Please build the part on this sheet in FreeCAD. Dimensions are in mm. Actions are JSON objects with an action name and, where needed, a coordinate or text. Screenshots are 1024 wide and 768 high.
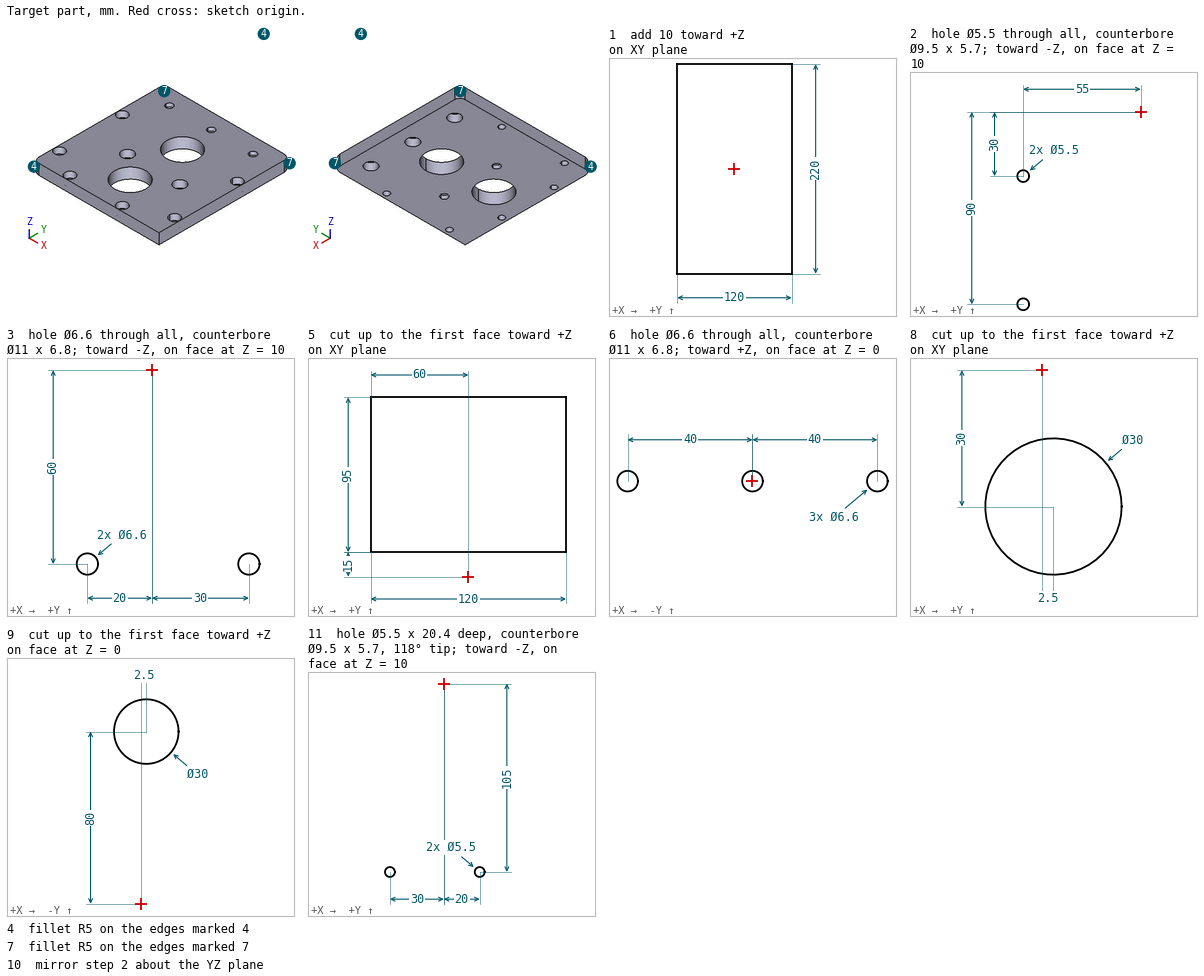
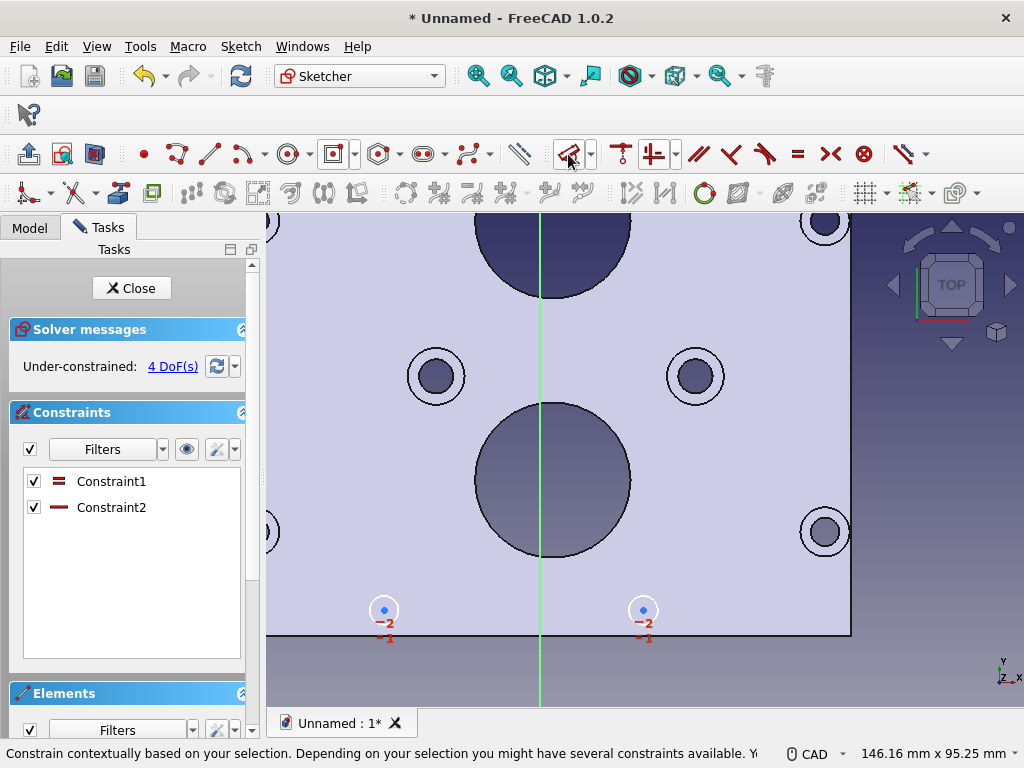
{"action": "scroll", "coordinate": [653, 600], "scroll_direction": "up", "scroll_amount": 2}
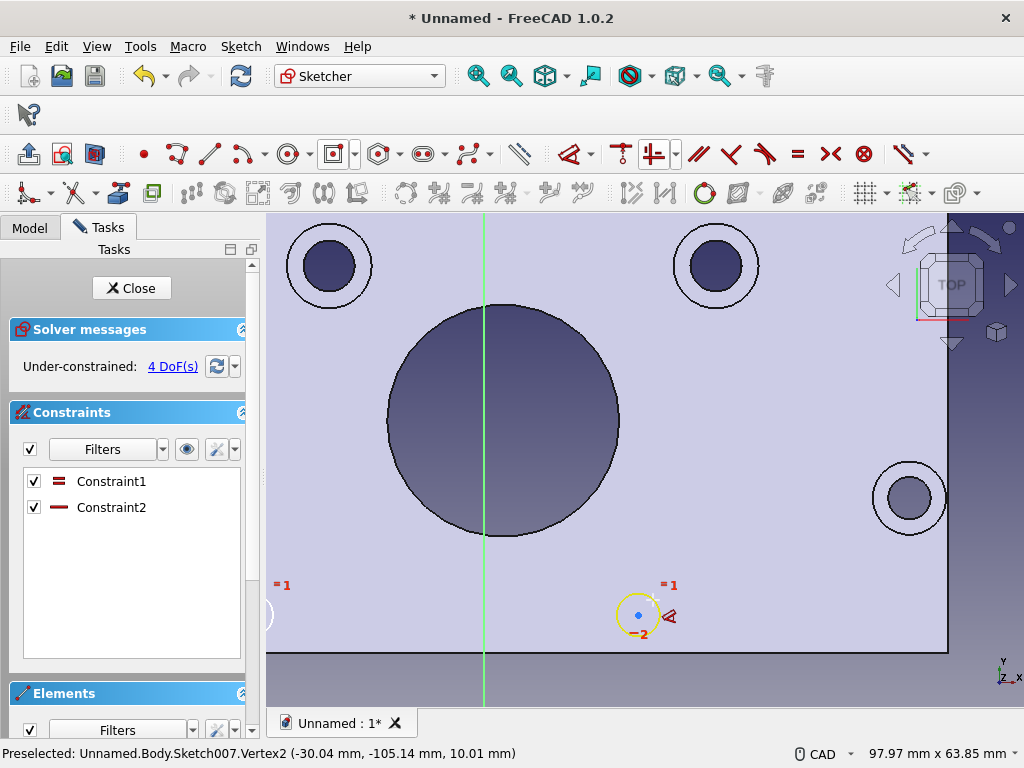
{"action": "left_click", "coordinate": [653, 600]}
{"action": "left_click", "coordinate": [675, 577]}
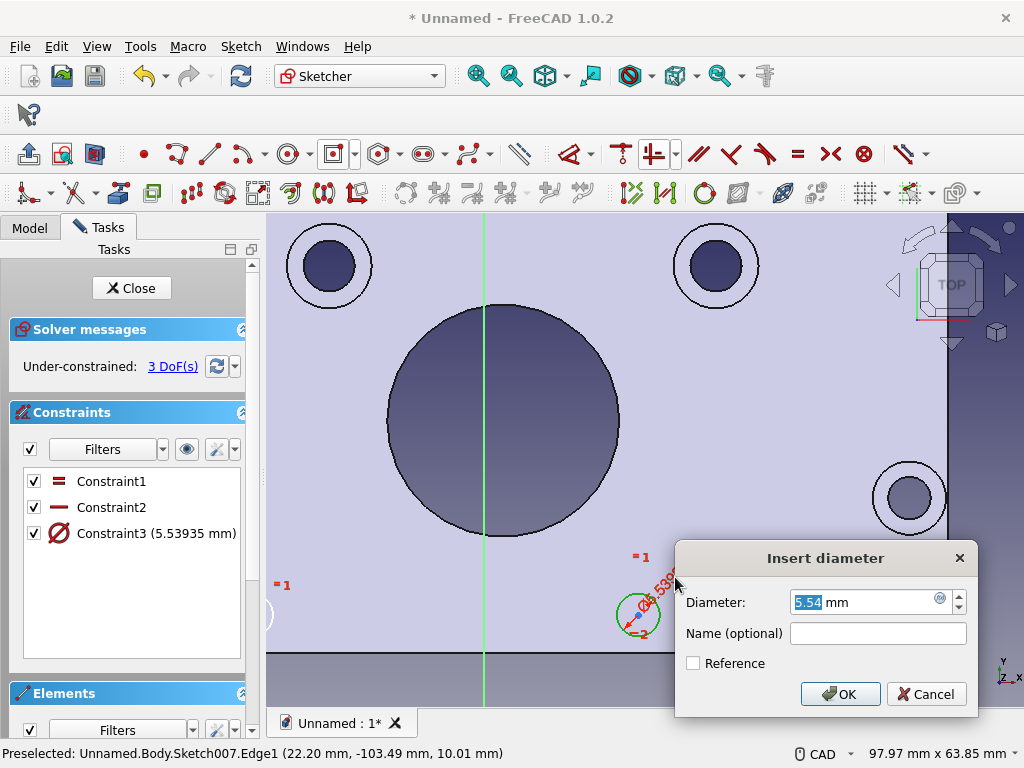
{"action": "type", "text": "5.5"}
{"action": "key", "text": "Return"}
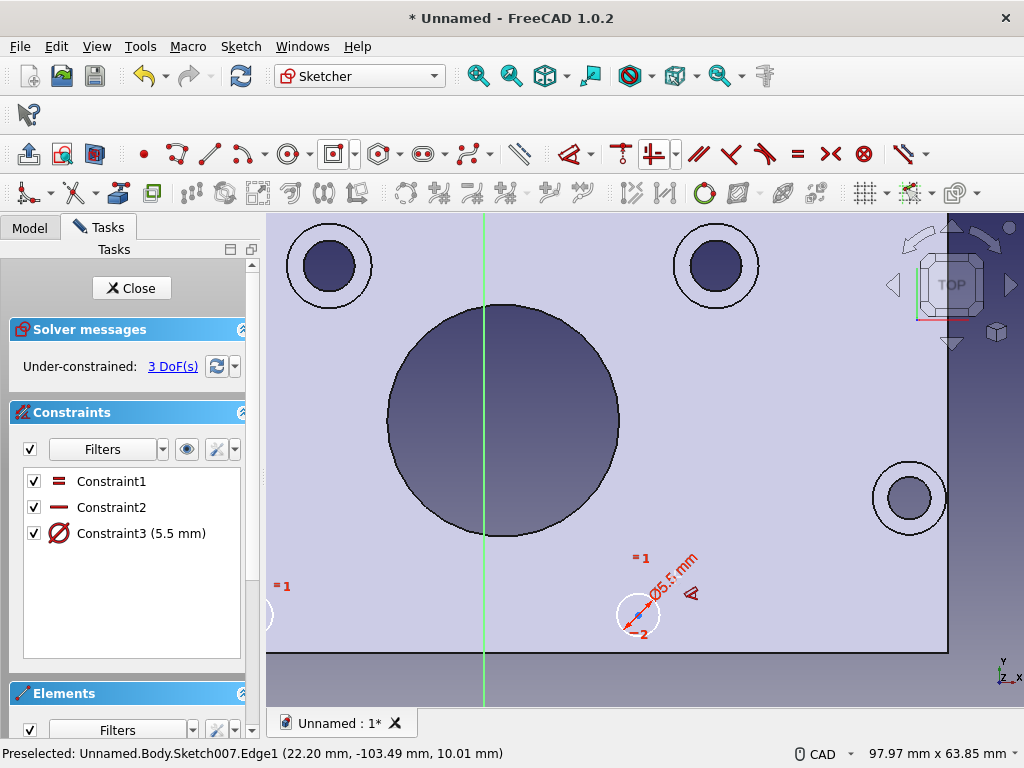
{"action": "left_click", "coordinate": [638, 615]}
{"action": "left_click", "coordinate": [561, 649]}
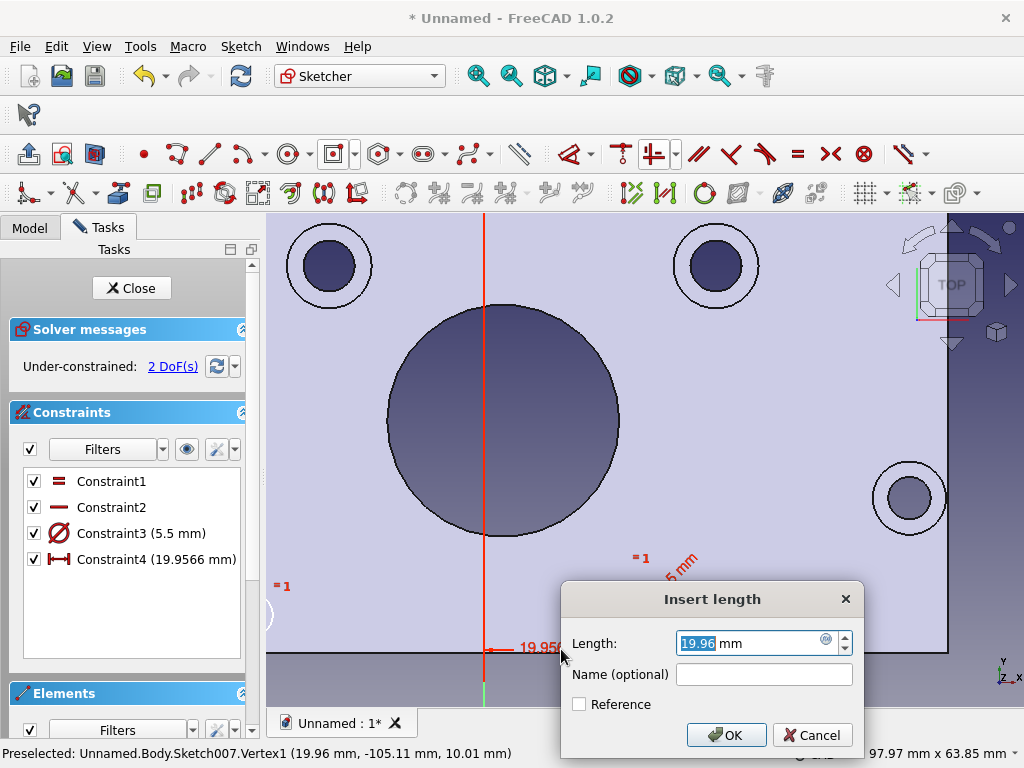
{"action": "type", "text": "20"}
{"action": "key", "text": "Return"}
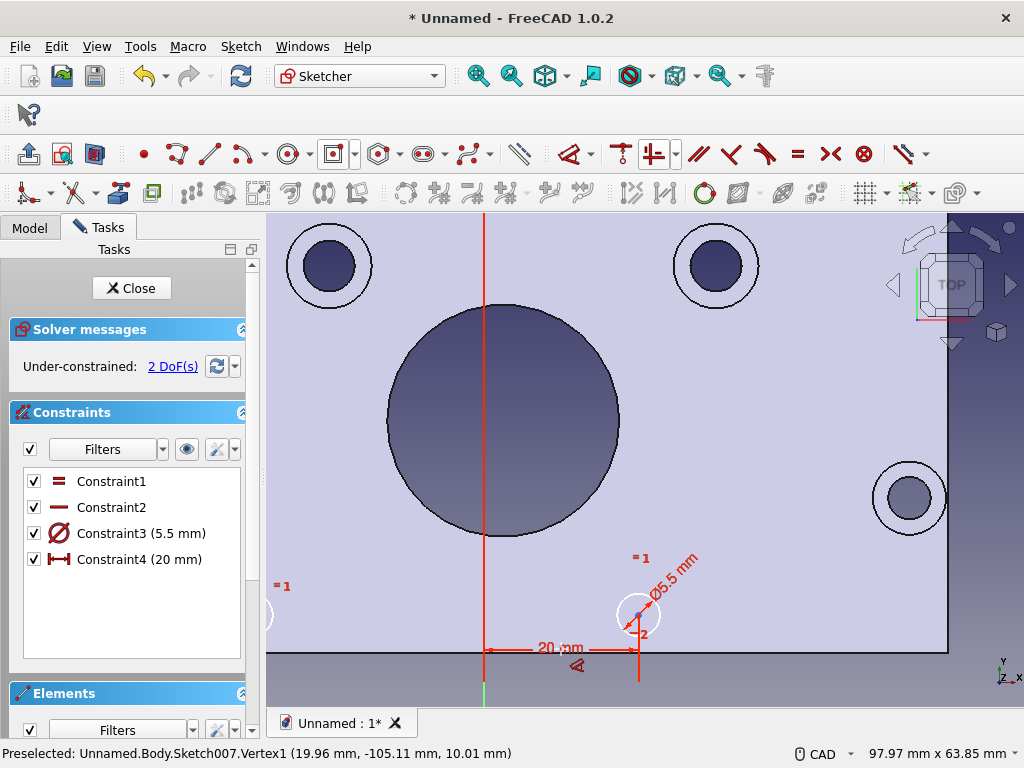
{"action": "scroll", "coordinate": [653, 600], "scroll_direction": "down", "scroll_amount": 5}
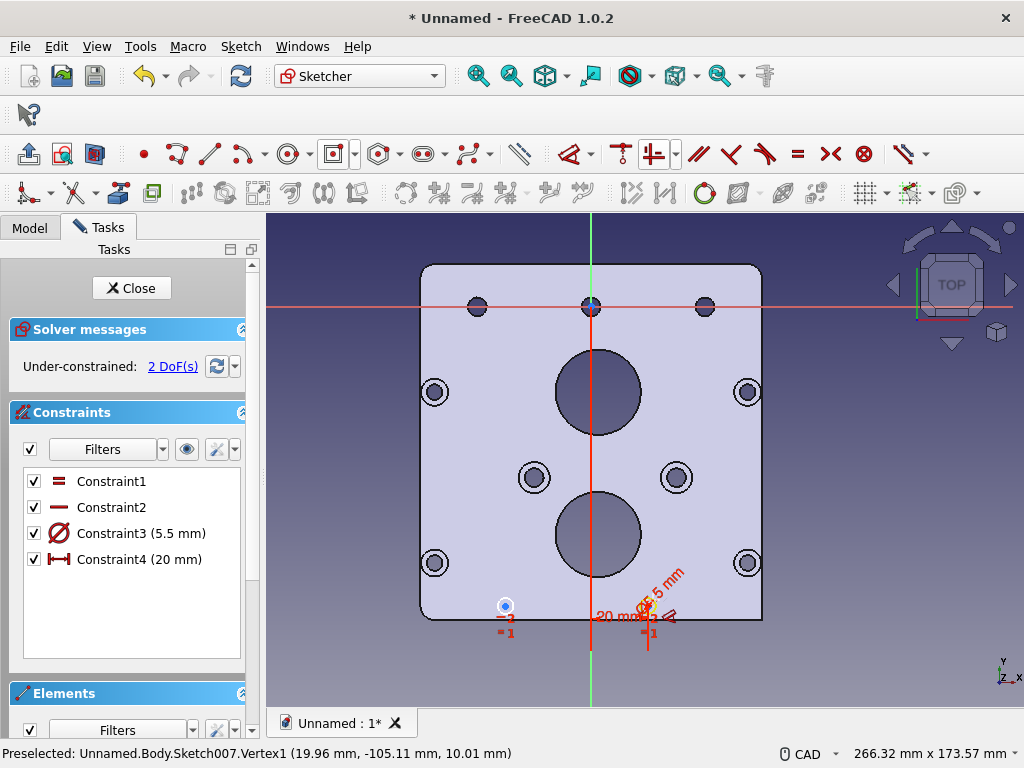
{"action": "left_click", "coordinate": [506, 606]}
{"action": "left_click", "coordinate": [548, 273]}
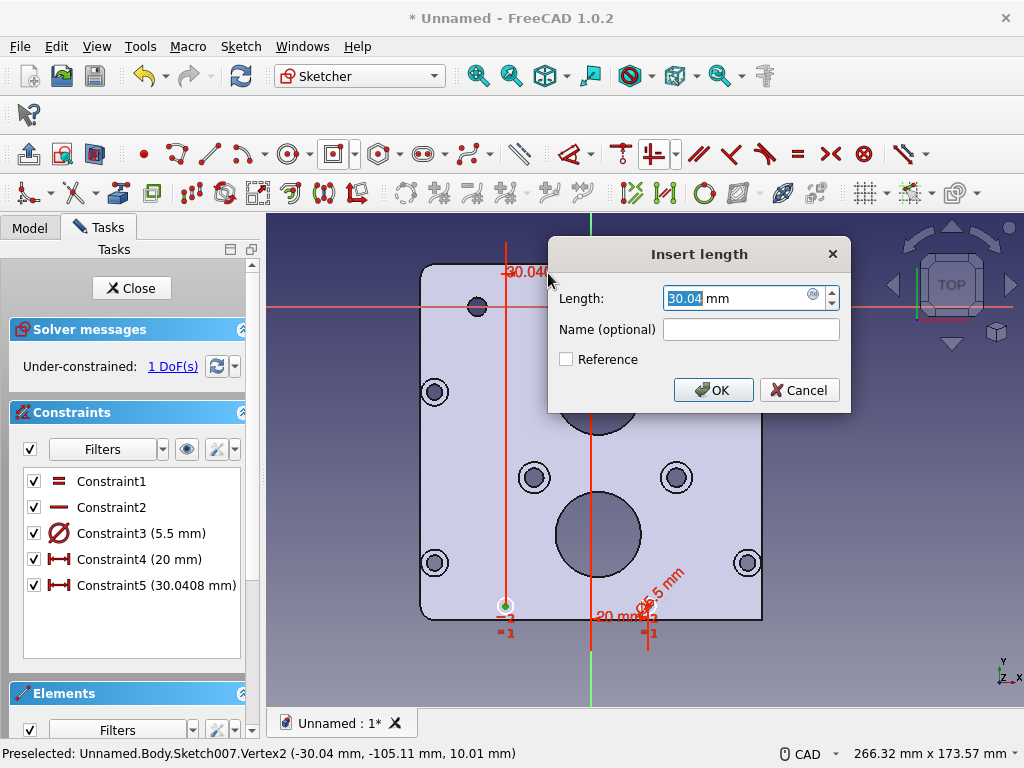
{"action": "type", "text": "30"}
{"action": "key", "text": "Return"}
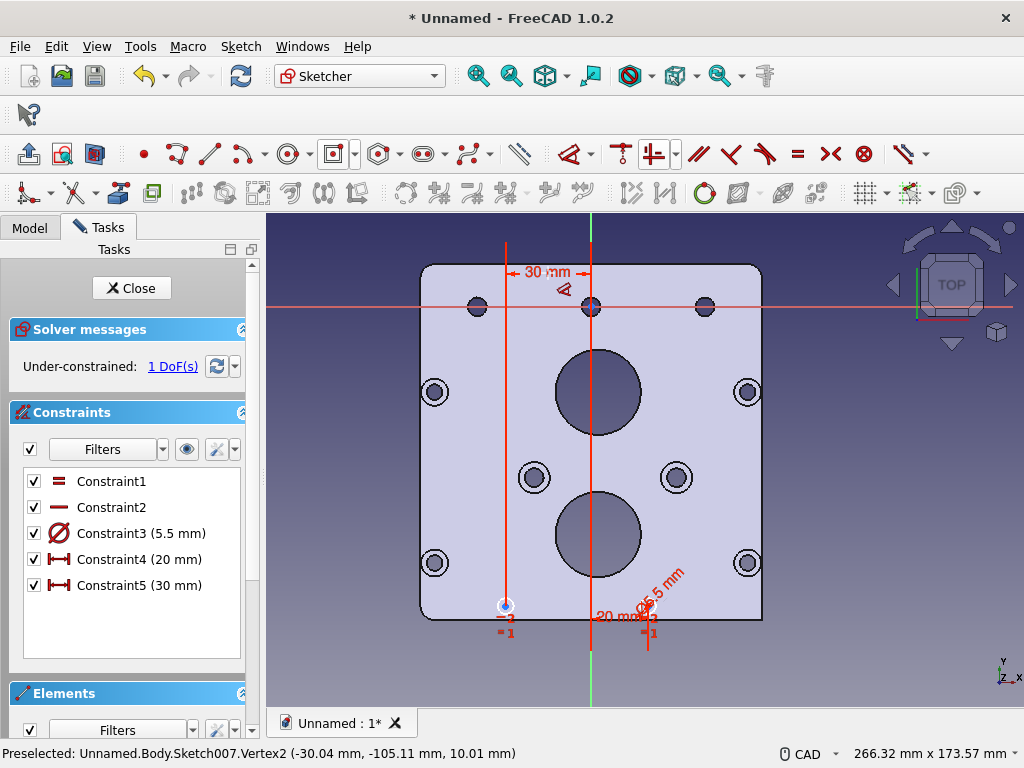
{"action": "left_click", "coordinate": [648, 606]}
{"action": "left_click", "coordinate": [682, 456]}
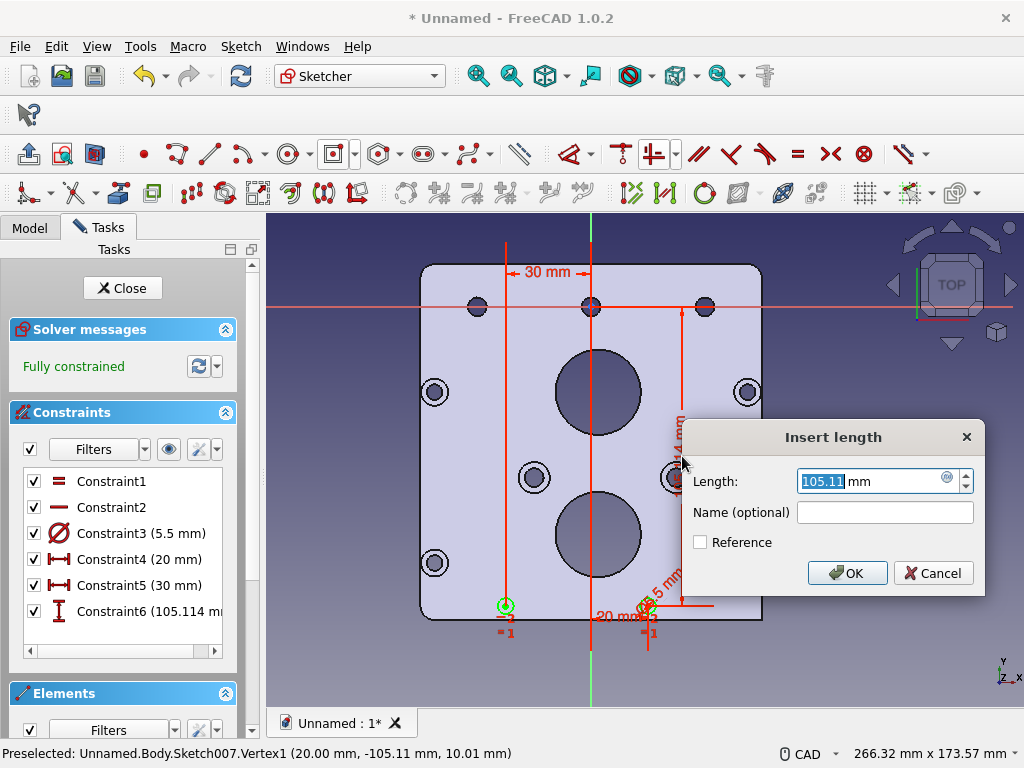
{"action": "type", "text": "105"}
{"action": "key", "text": "Return"}
{"action": "key", "text": "Escape"}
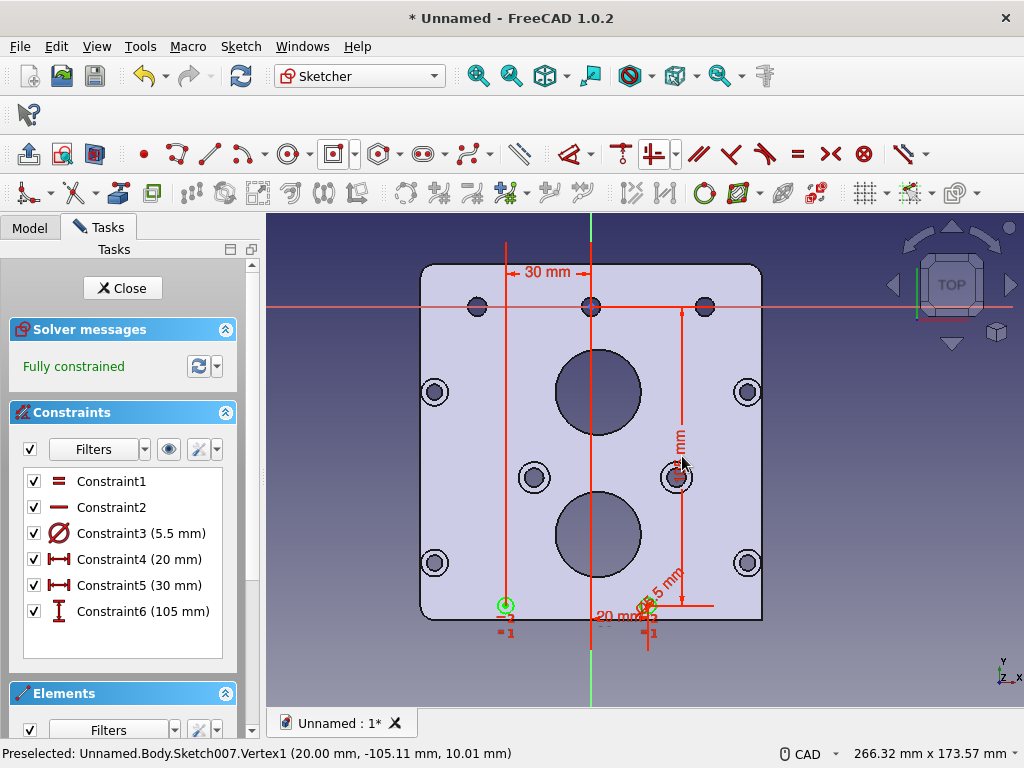
{"action": "left_click", "coordinate": [123, 288]}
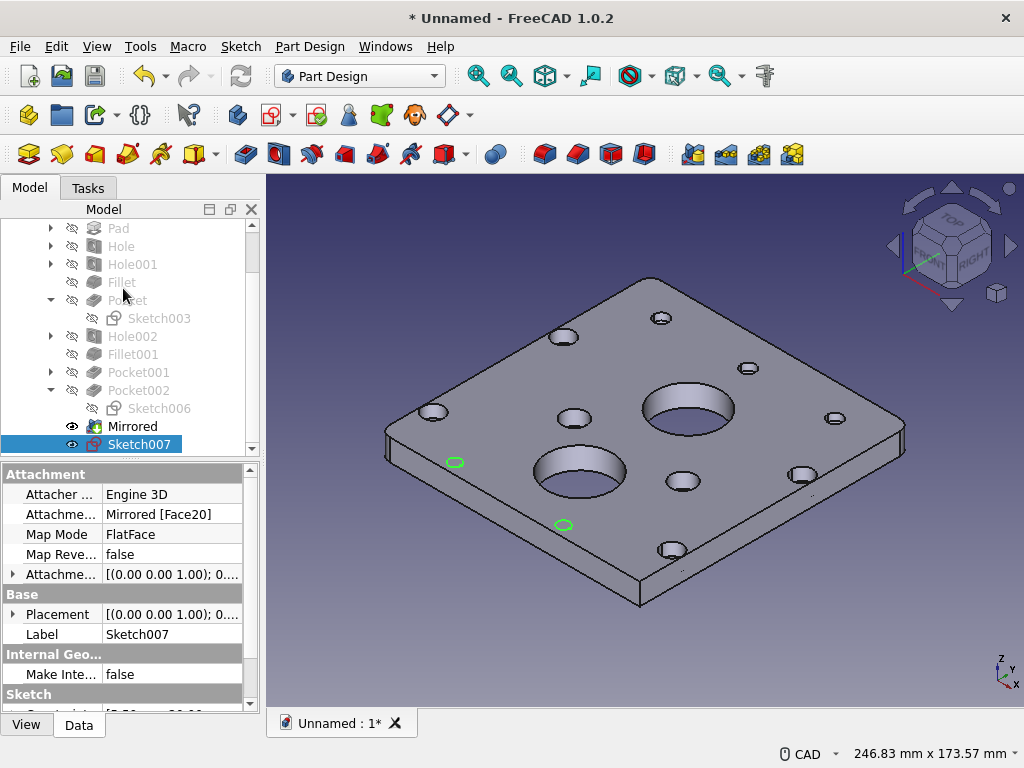
{"action": "left_click", "coordinate": [279, 154]}